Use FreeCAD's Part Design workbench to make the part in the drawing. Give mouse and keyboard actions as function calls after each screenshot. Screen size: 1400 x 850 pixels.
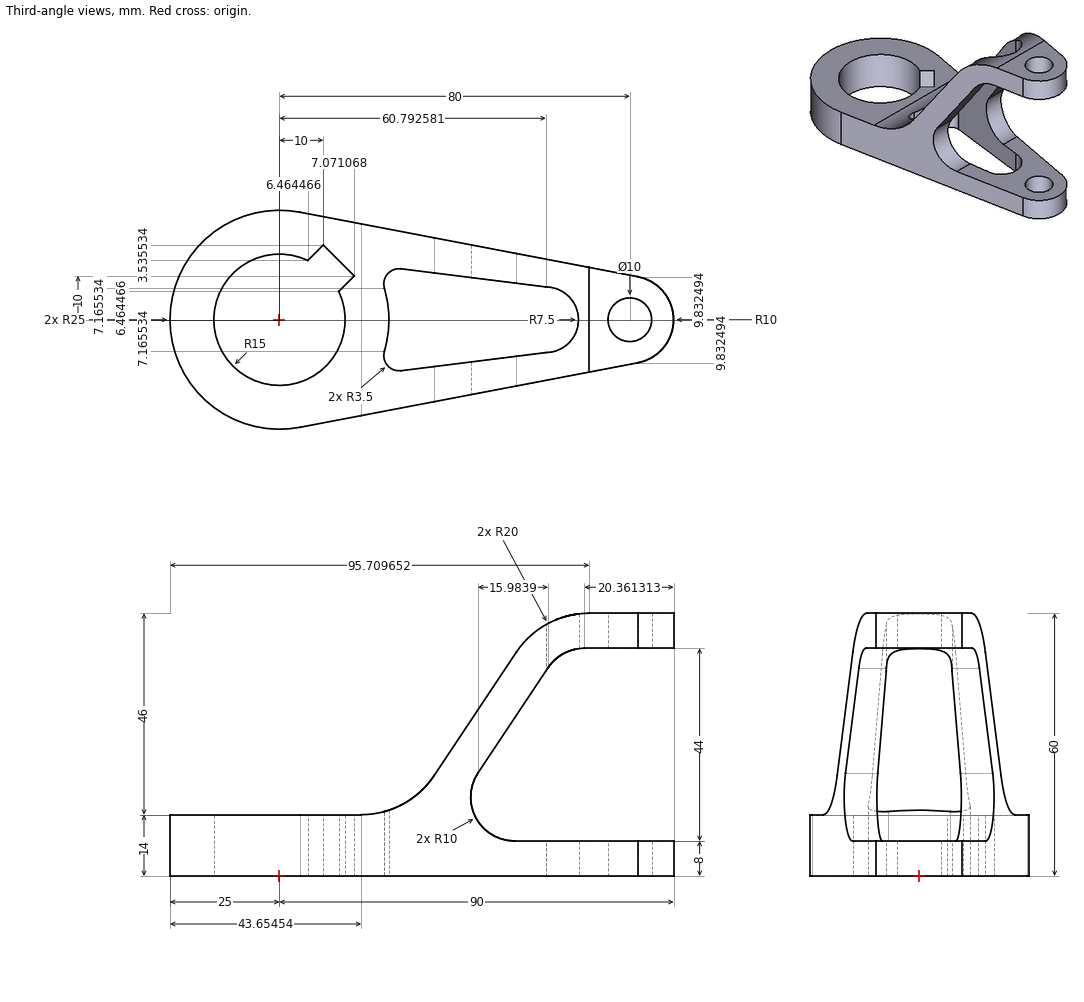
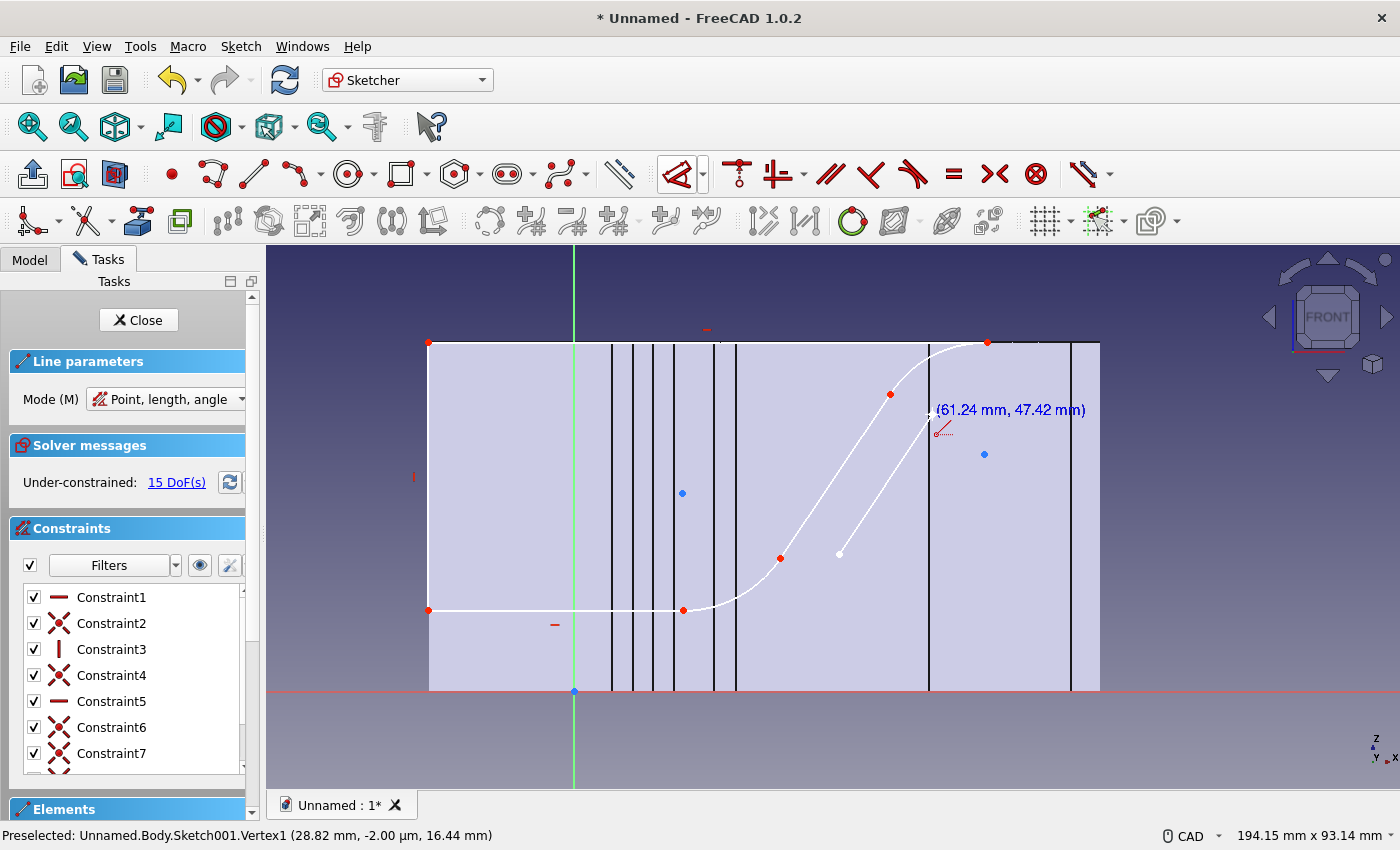
click(213, 174)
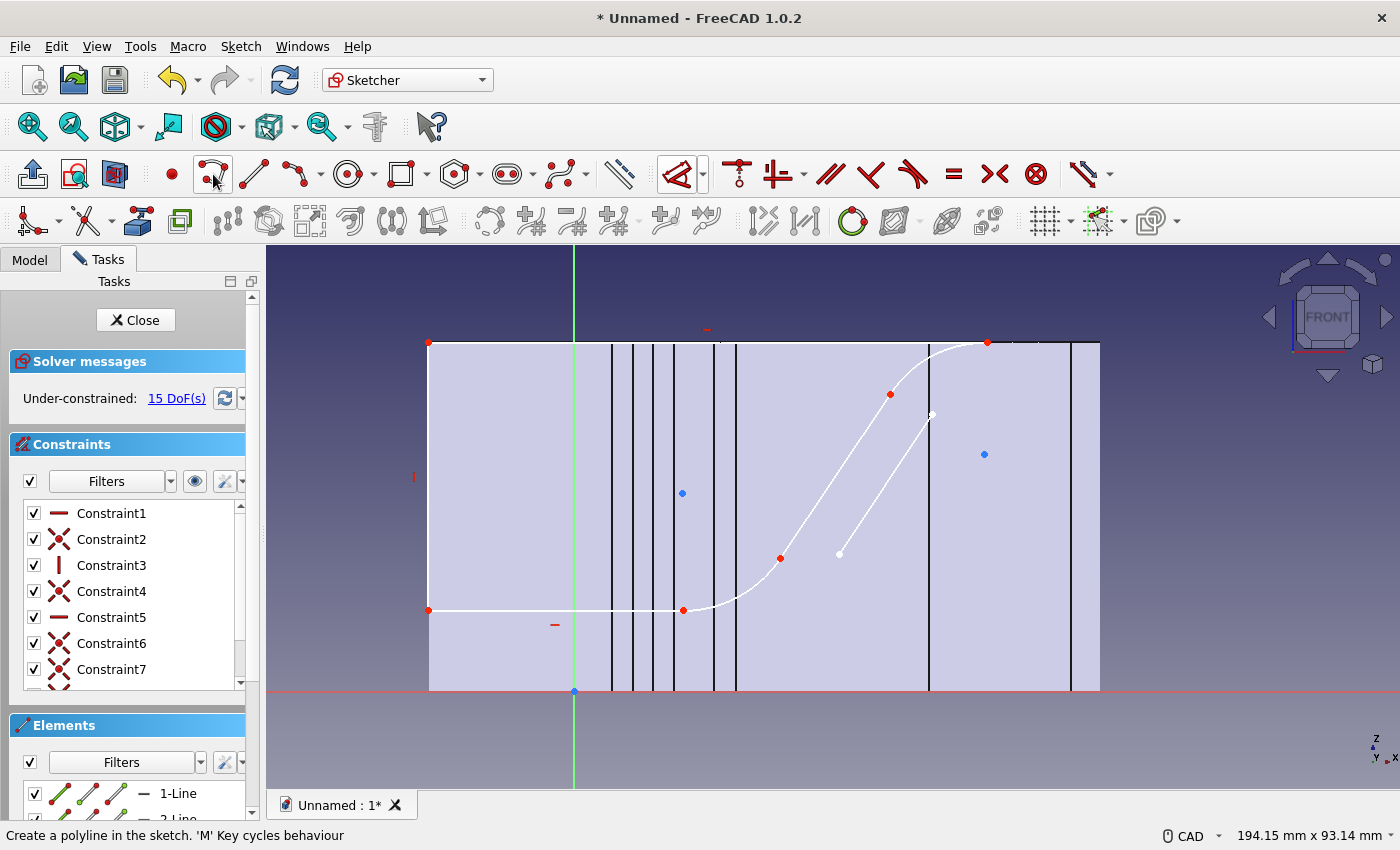
click(981, 388)
click(1100, 388)
click(1100, 645)
click(888, 645)
right_click(888, 645)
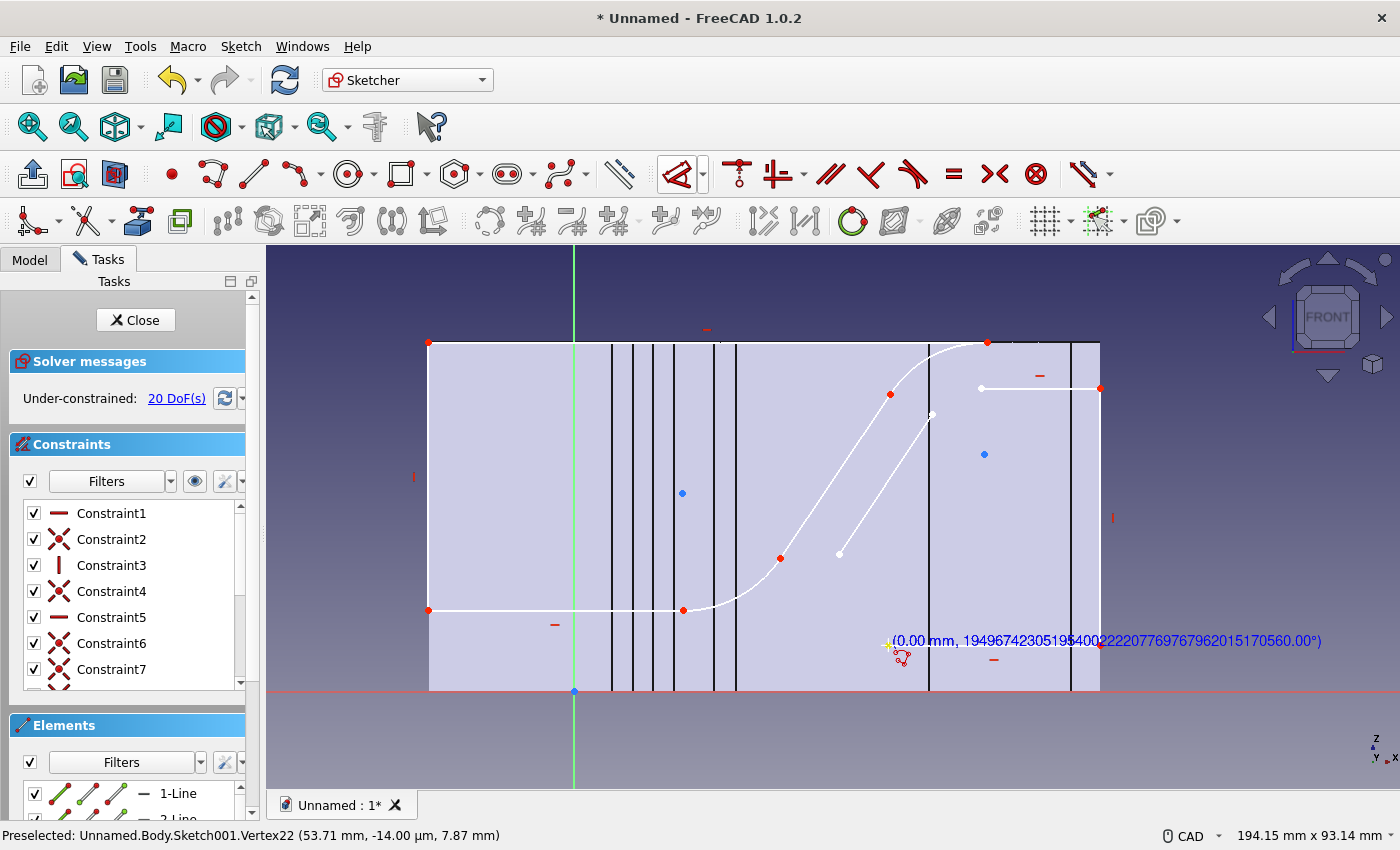
key(g)
key(3)
key(a)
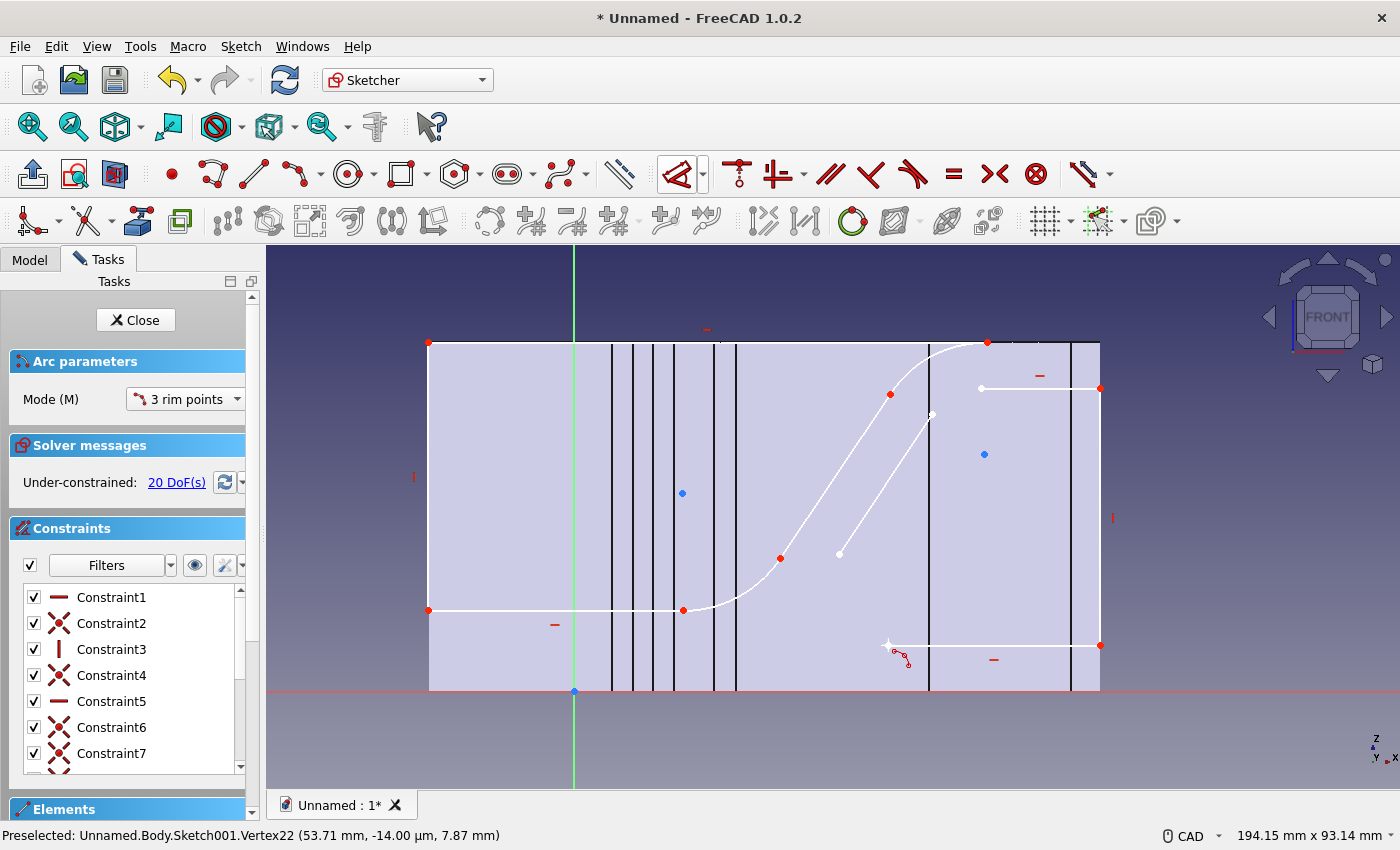
click(932, 415)
click(981, 389)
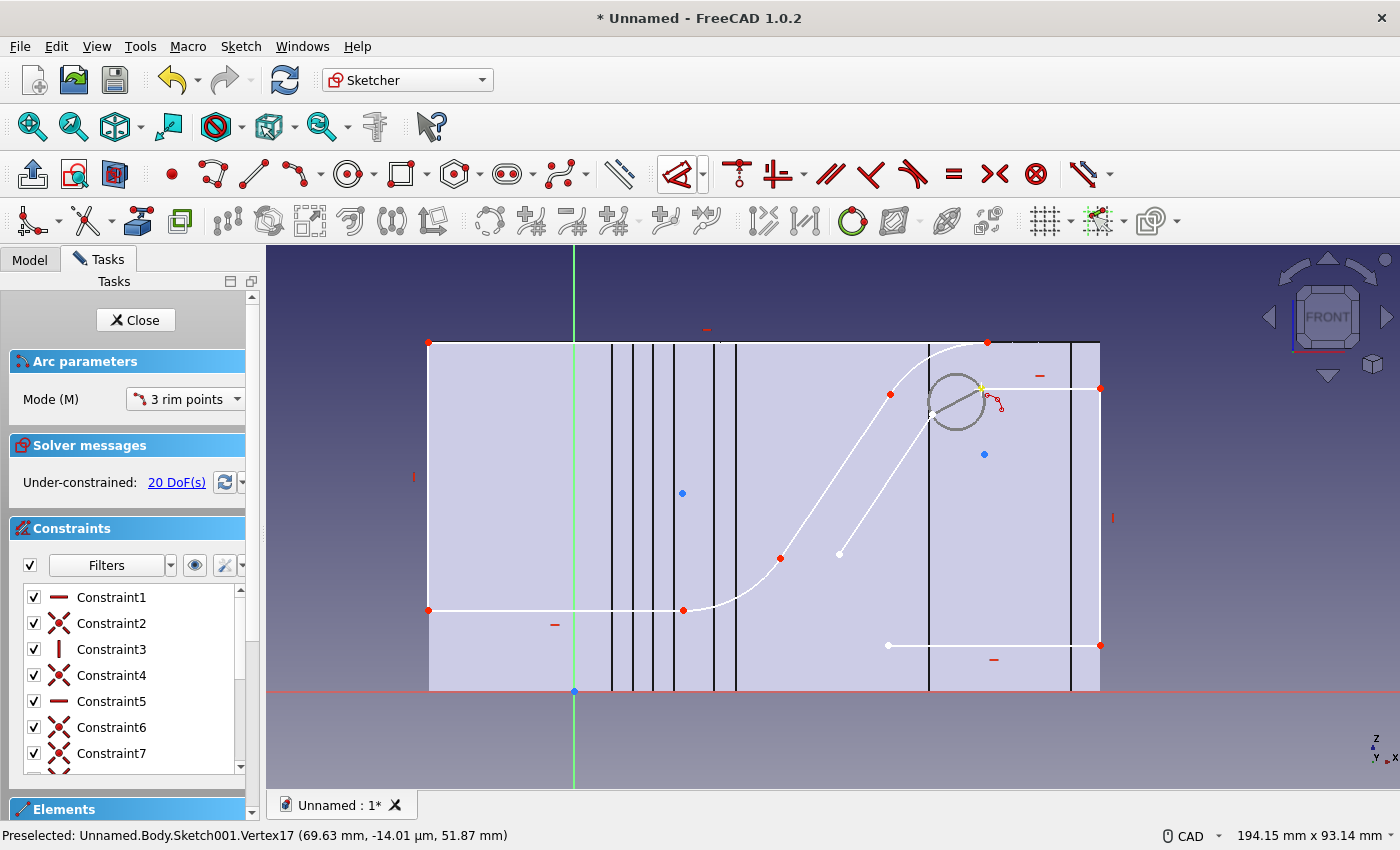
scroll(953, 395, up, 5)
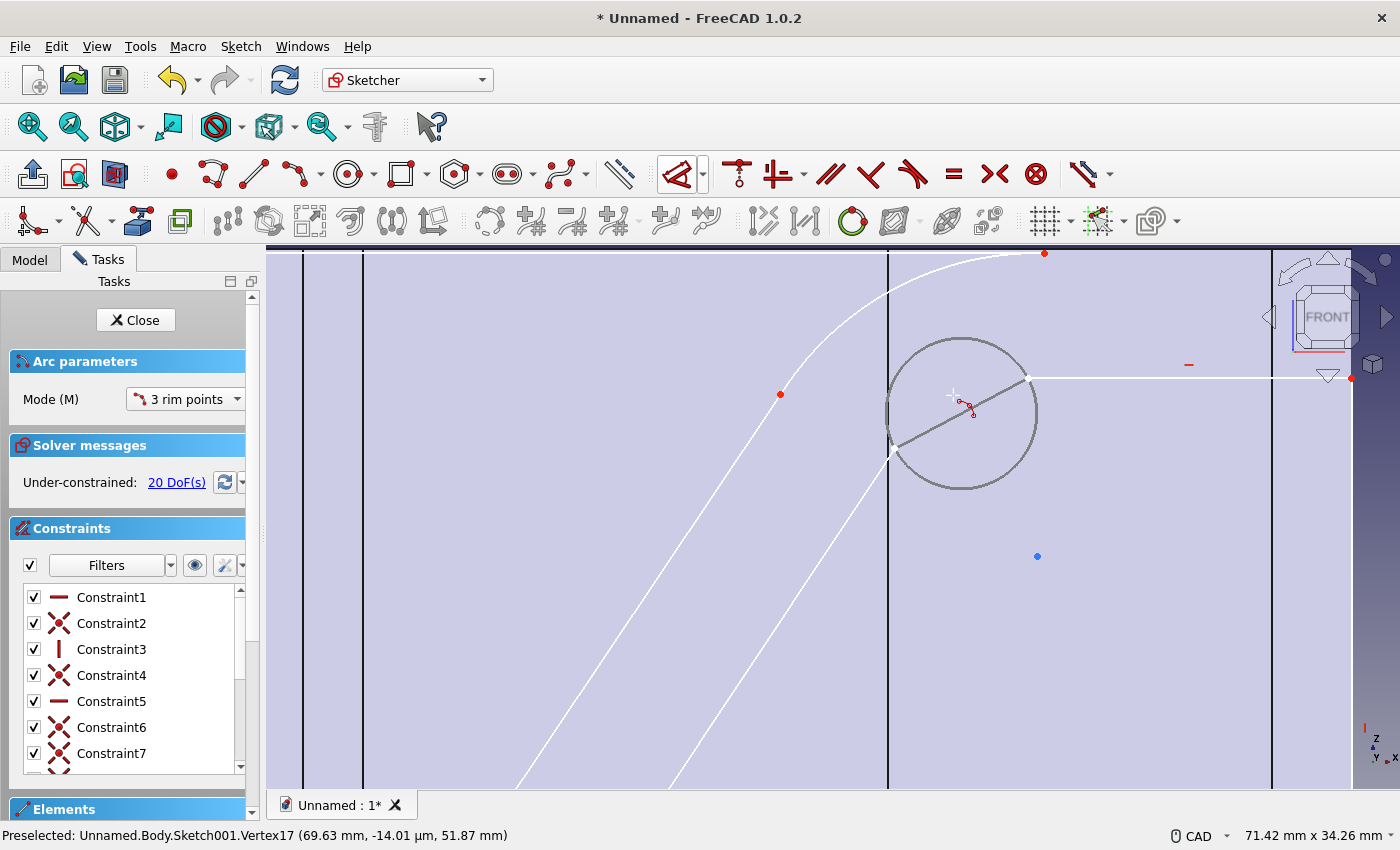
click(953, 395)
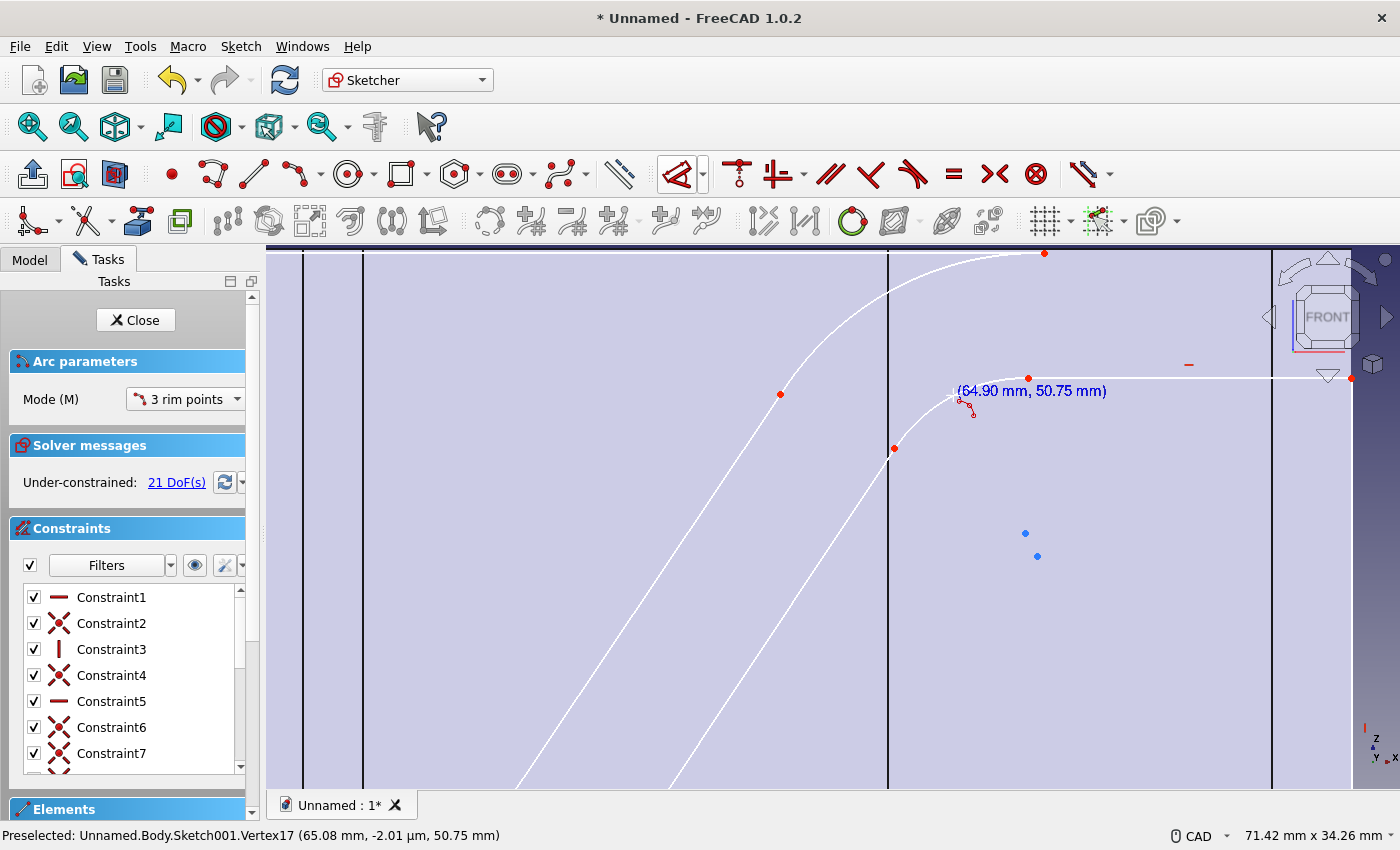
scroll(954, 396, down, 5)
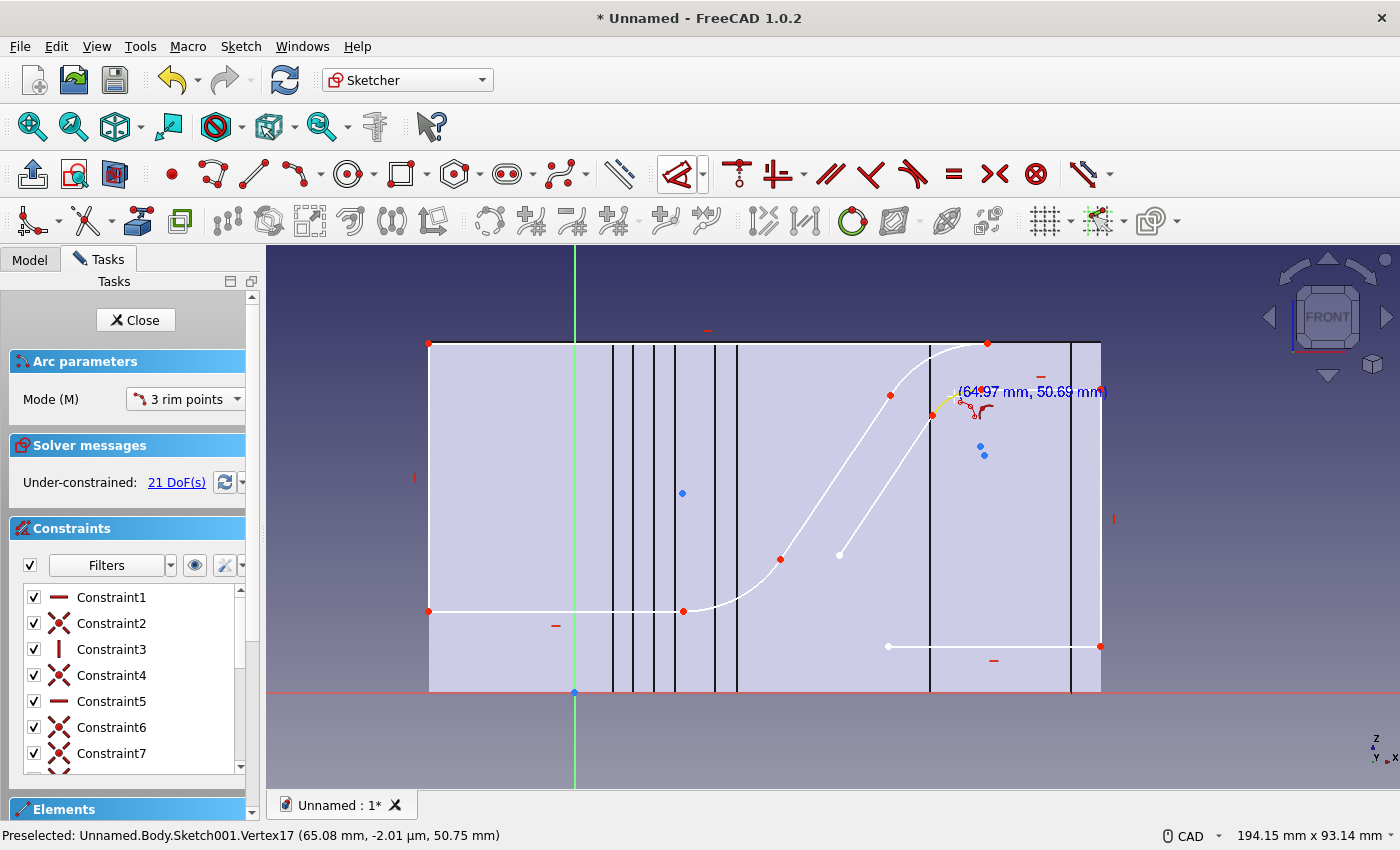
click(889, 647)
click(840, 556)
click(837, 615)
key(Escape)